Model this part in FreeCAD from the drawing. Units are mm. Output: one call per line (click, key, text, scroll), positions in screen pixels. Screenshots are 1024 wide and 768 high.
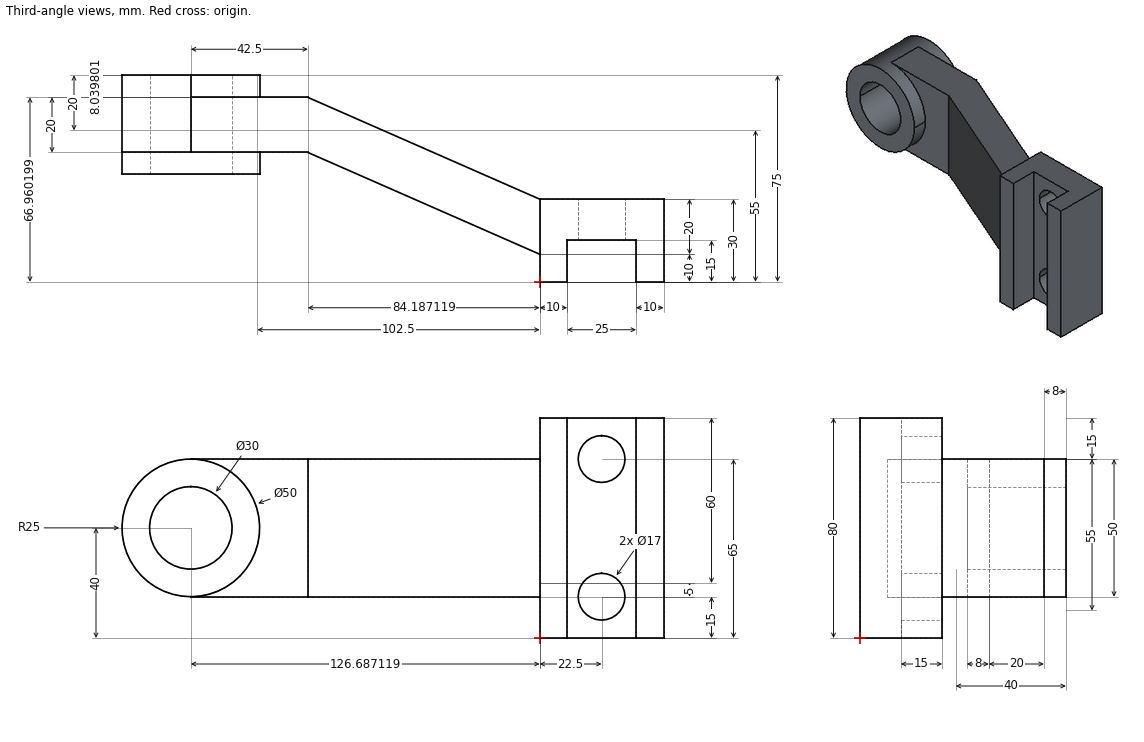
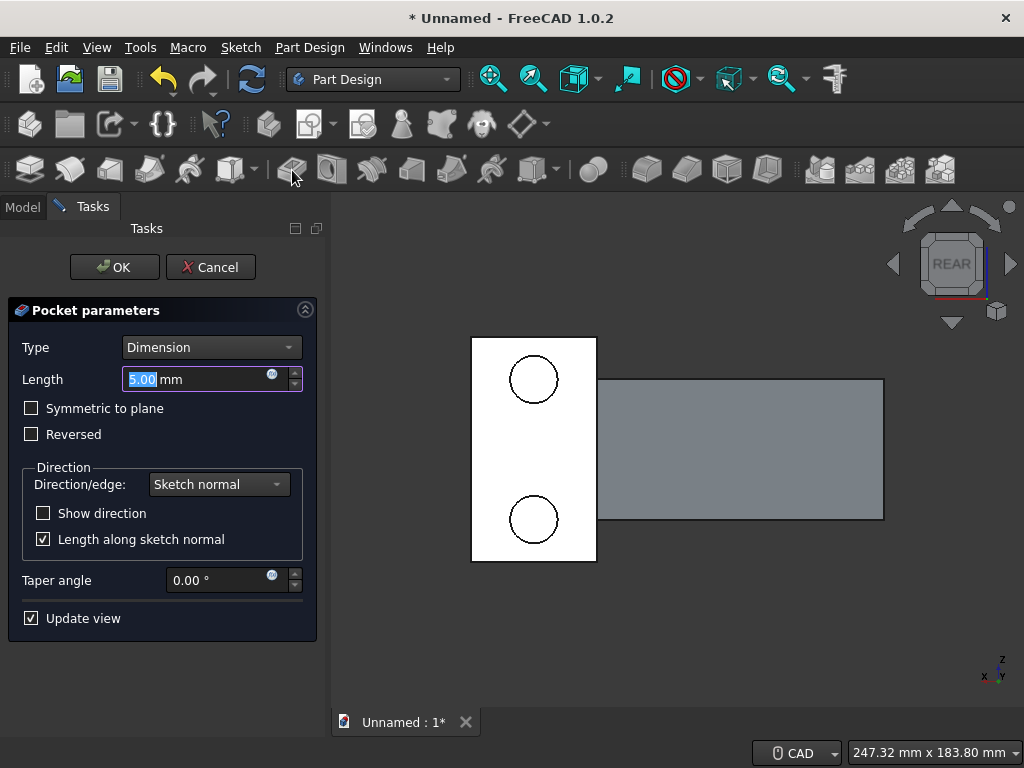
text(15)
key(Tab)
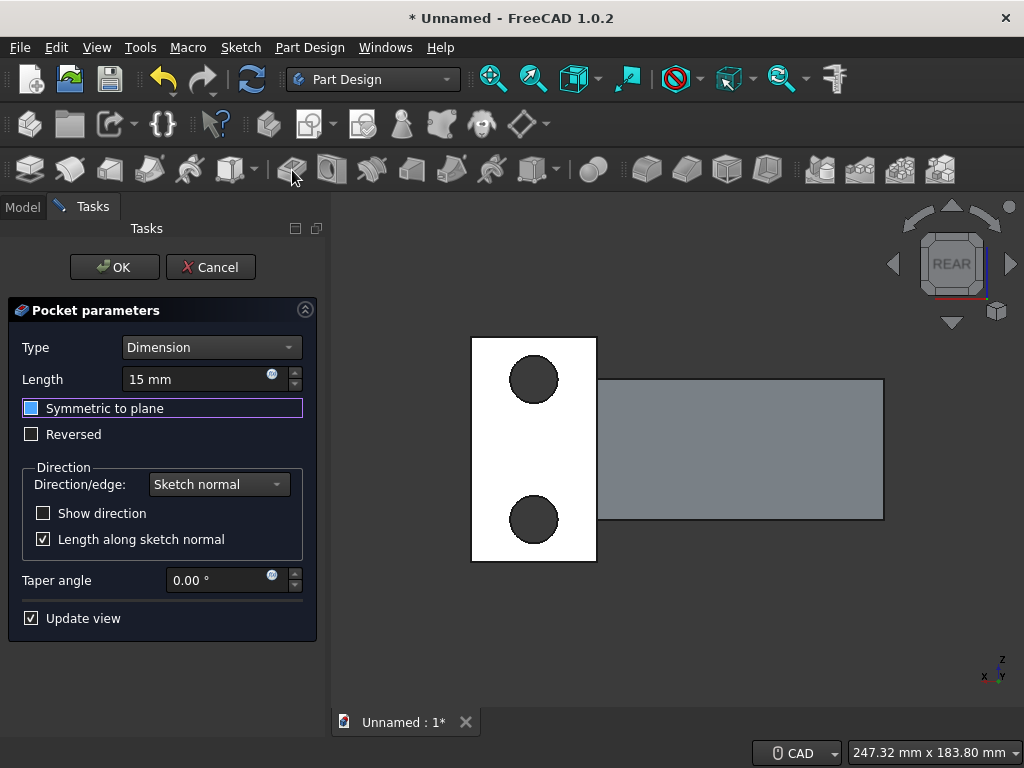
click(115, 267)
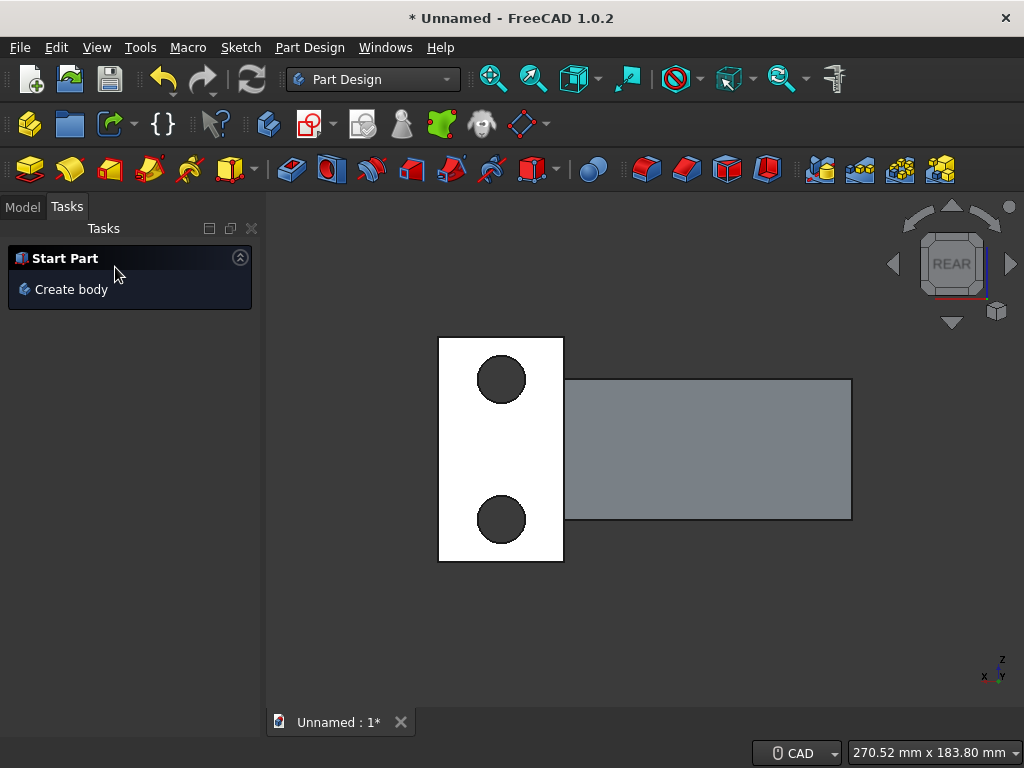
key(0)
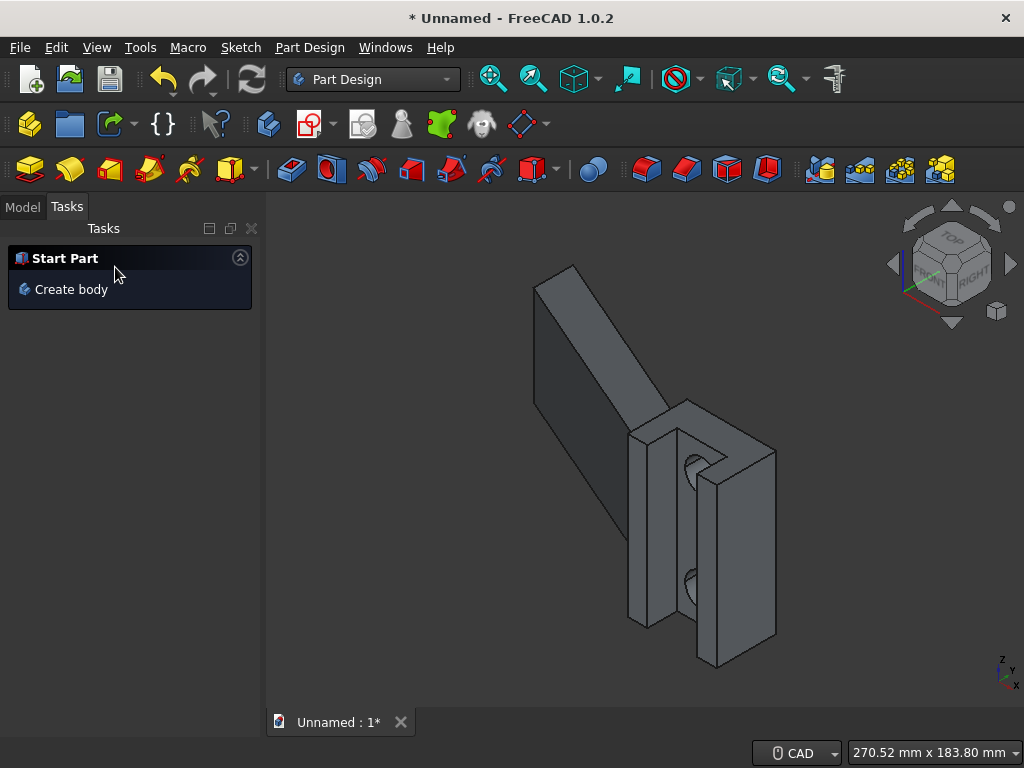
click(610, 360)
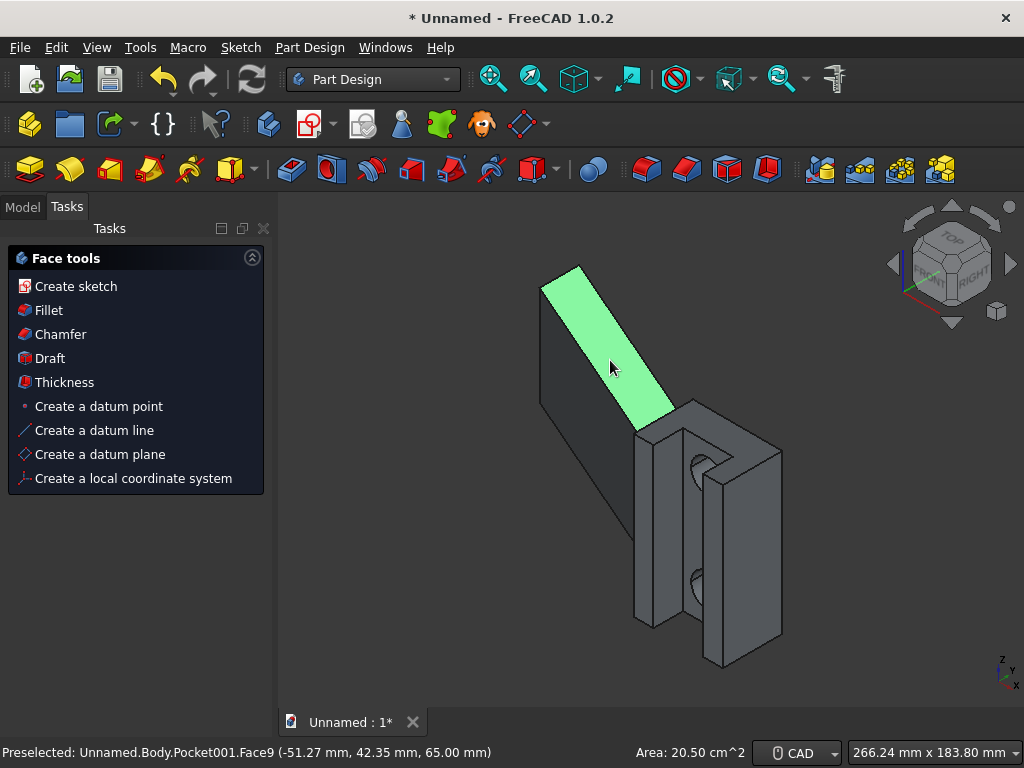
click(310, 124)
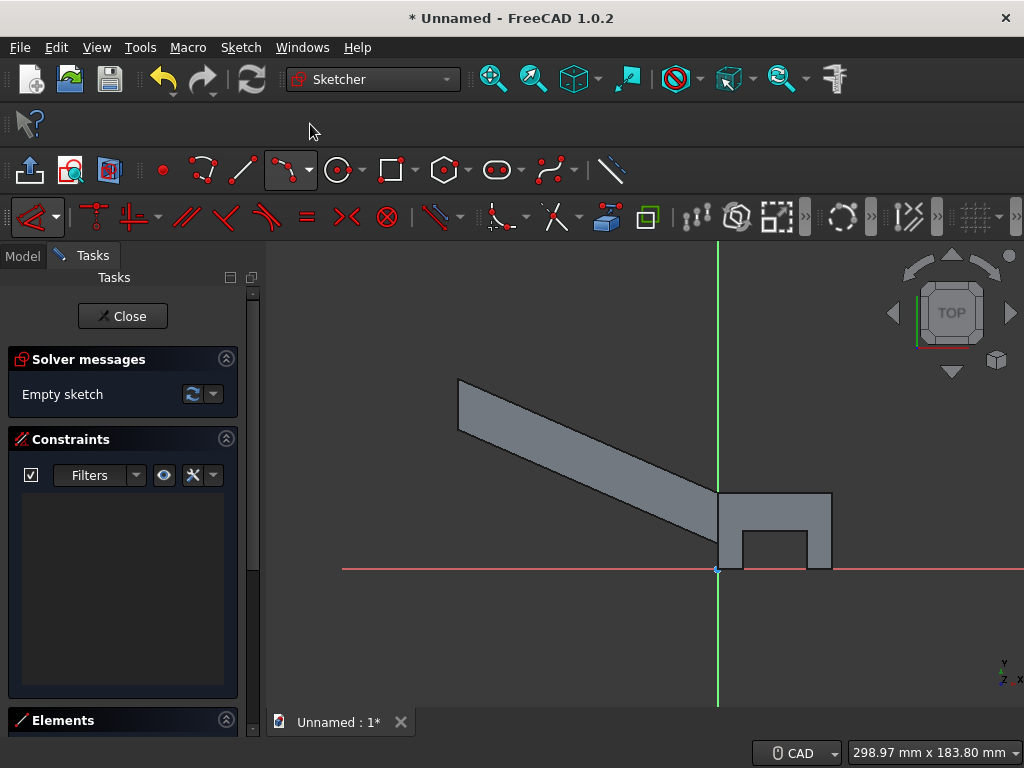
key(q)
key(s)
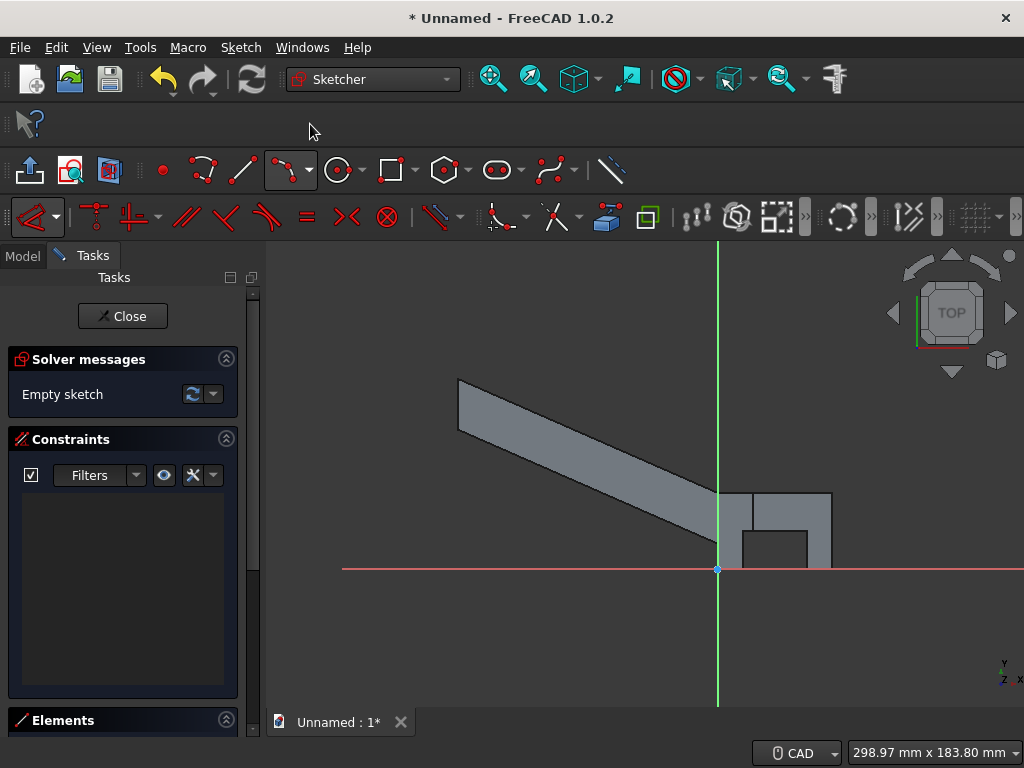
scroll(450, 395, up, 7)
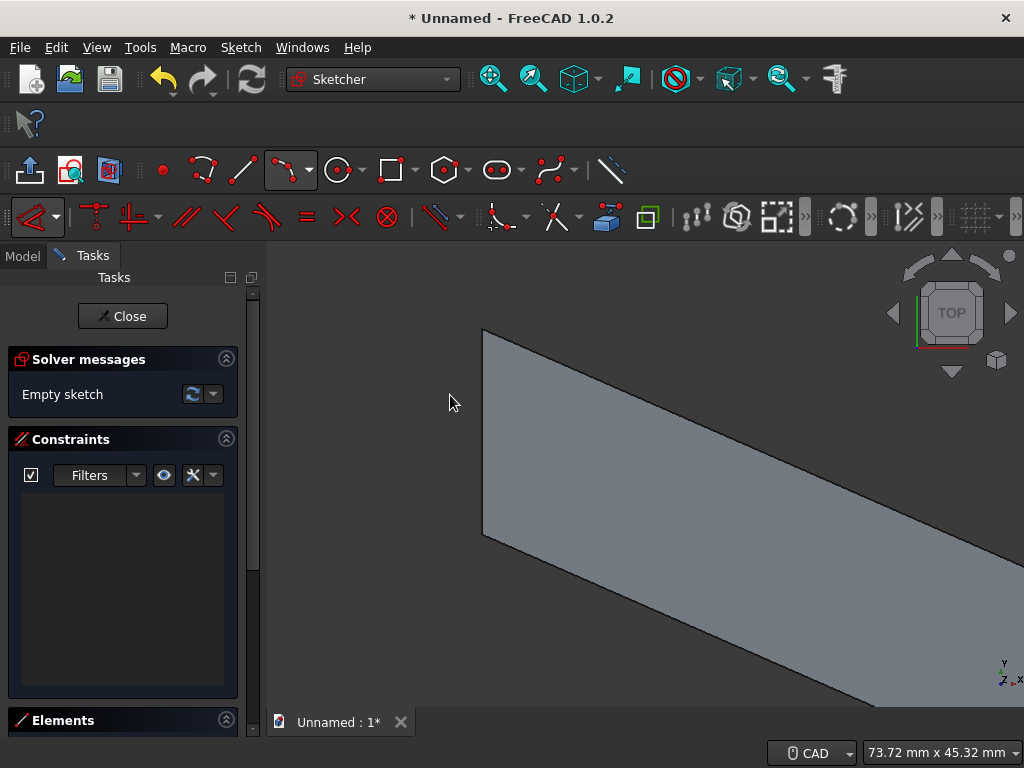
click(204, 170)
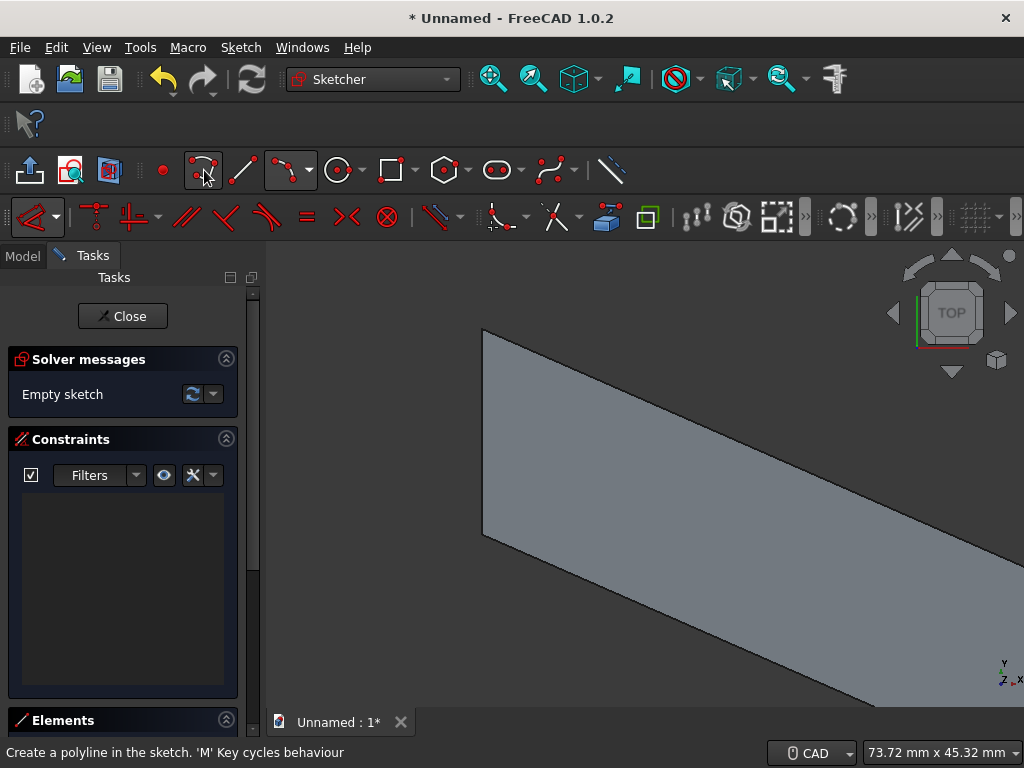
click(670, 617)
click(670, 411)
click(482, 329)
click(482, 534)
click(670, 618)
key(Escape)
key(Escape)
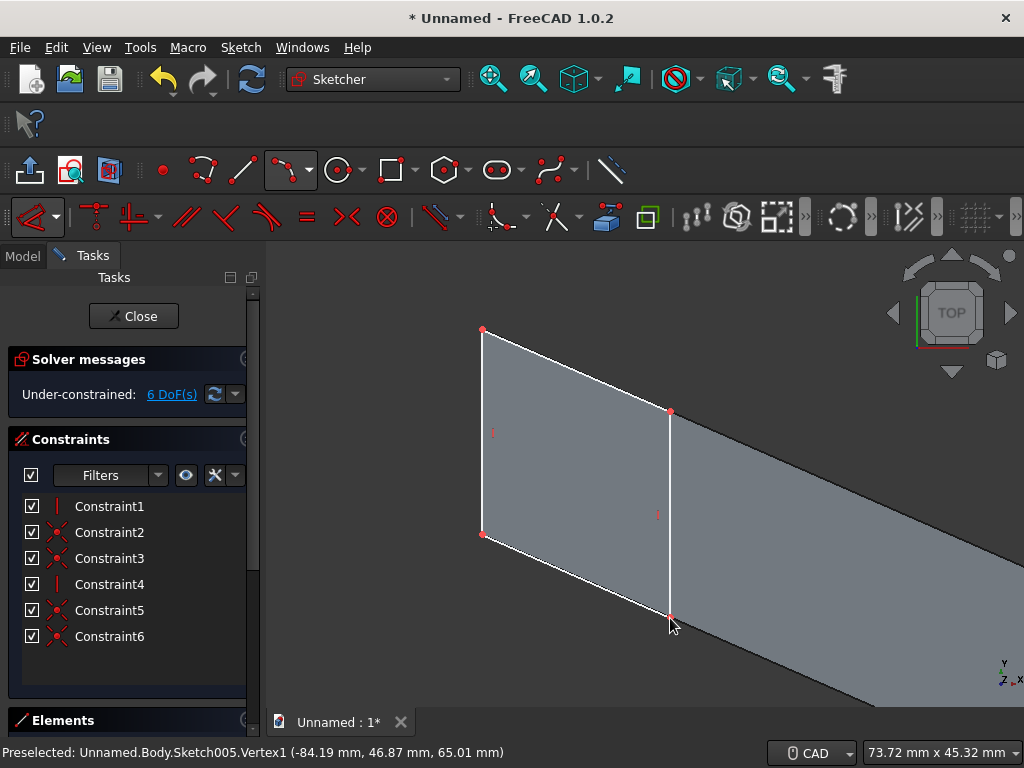
click(670, 556)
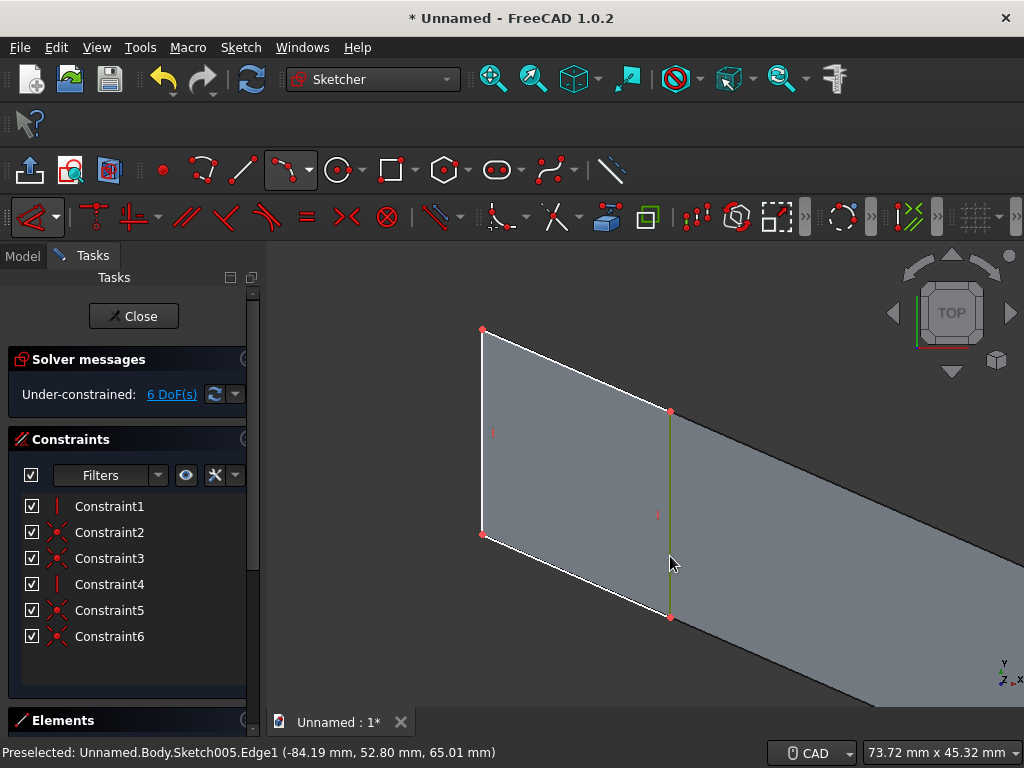
key(i)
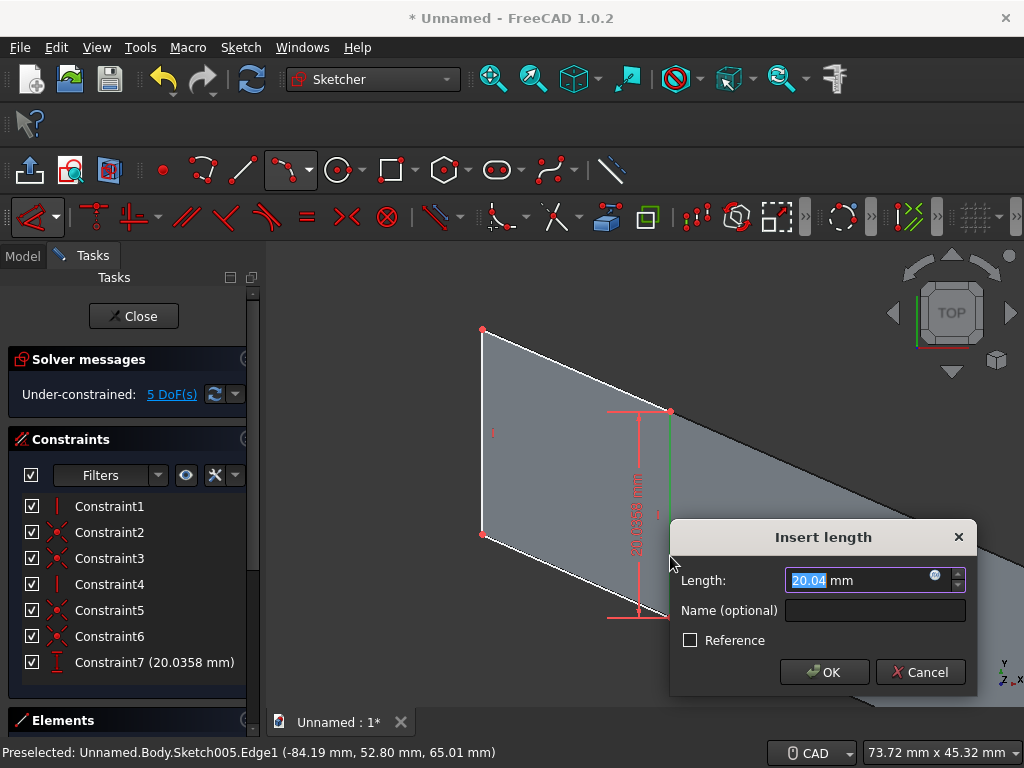
text(20)
key(Return)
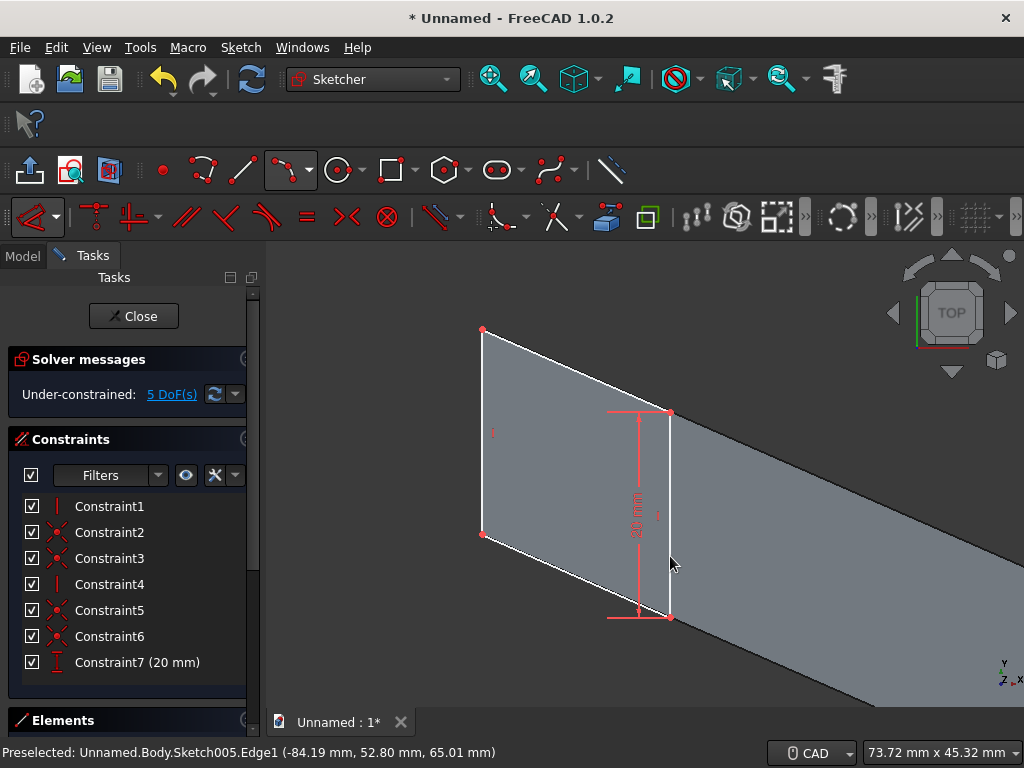
click(482, 392)